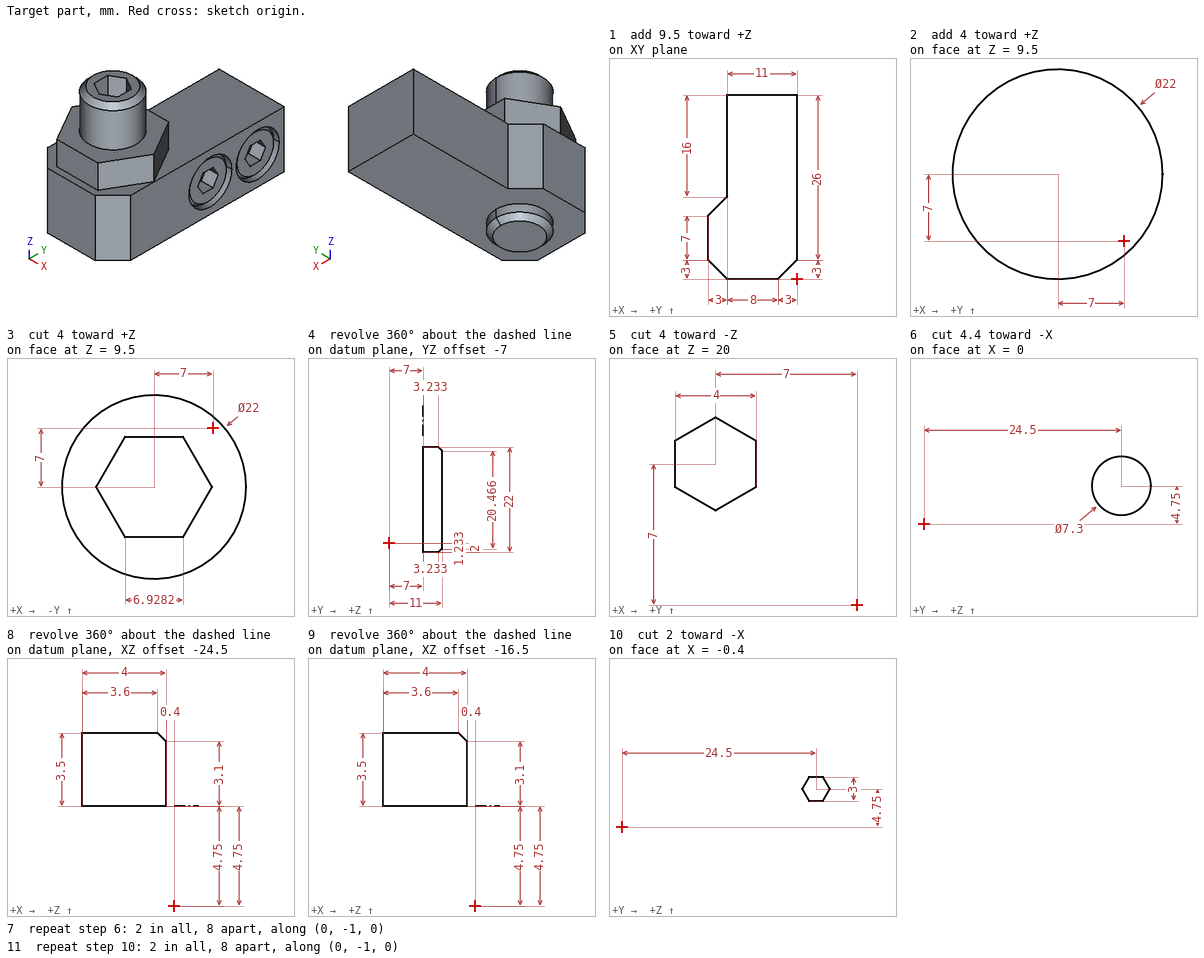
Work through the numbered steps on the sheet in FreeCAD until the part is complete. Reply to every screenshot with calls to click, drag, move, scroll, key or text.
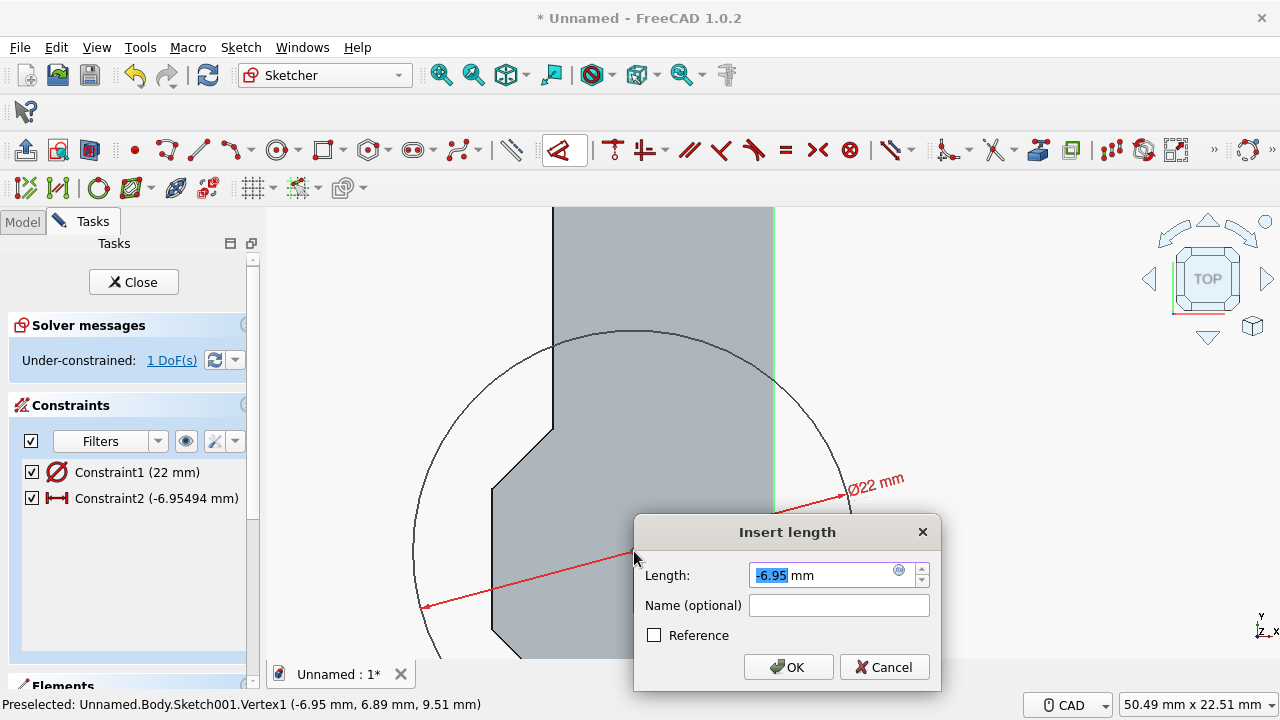
text(-7)
key(Return)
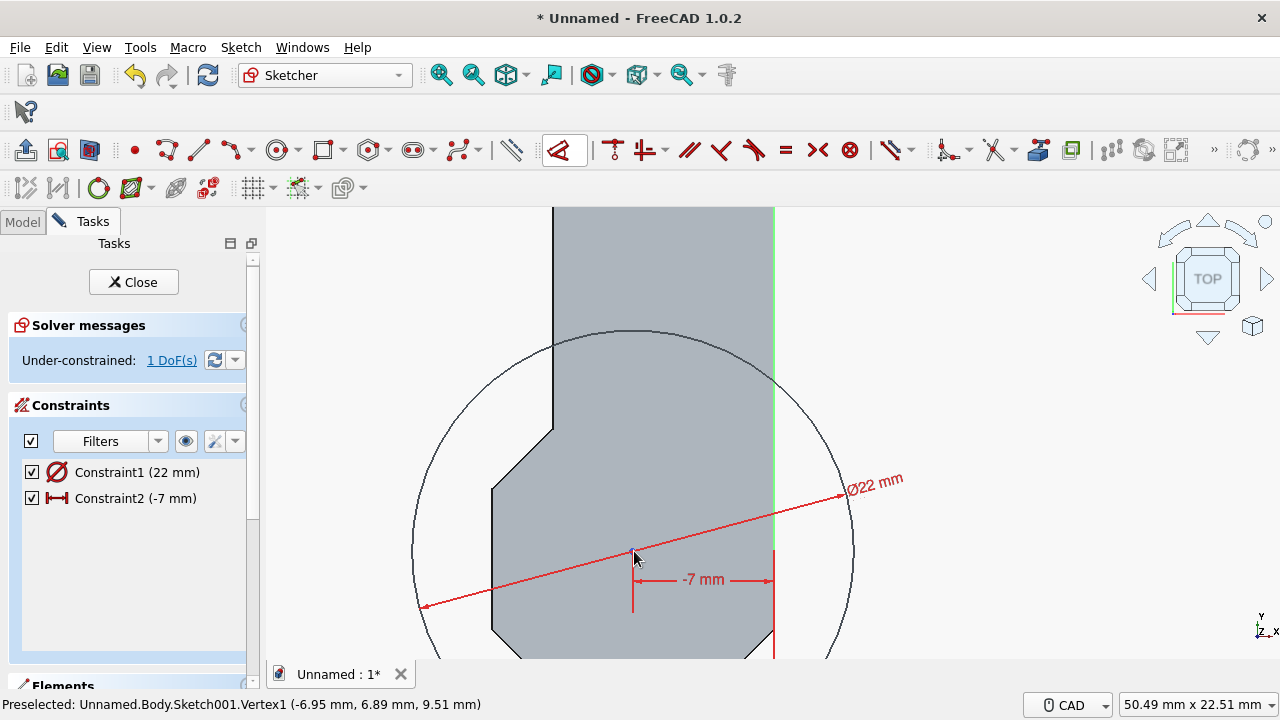
click(633, 551)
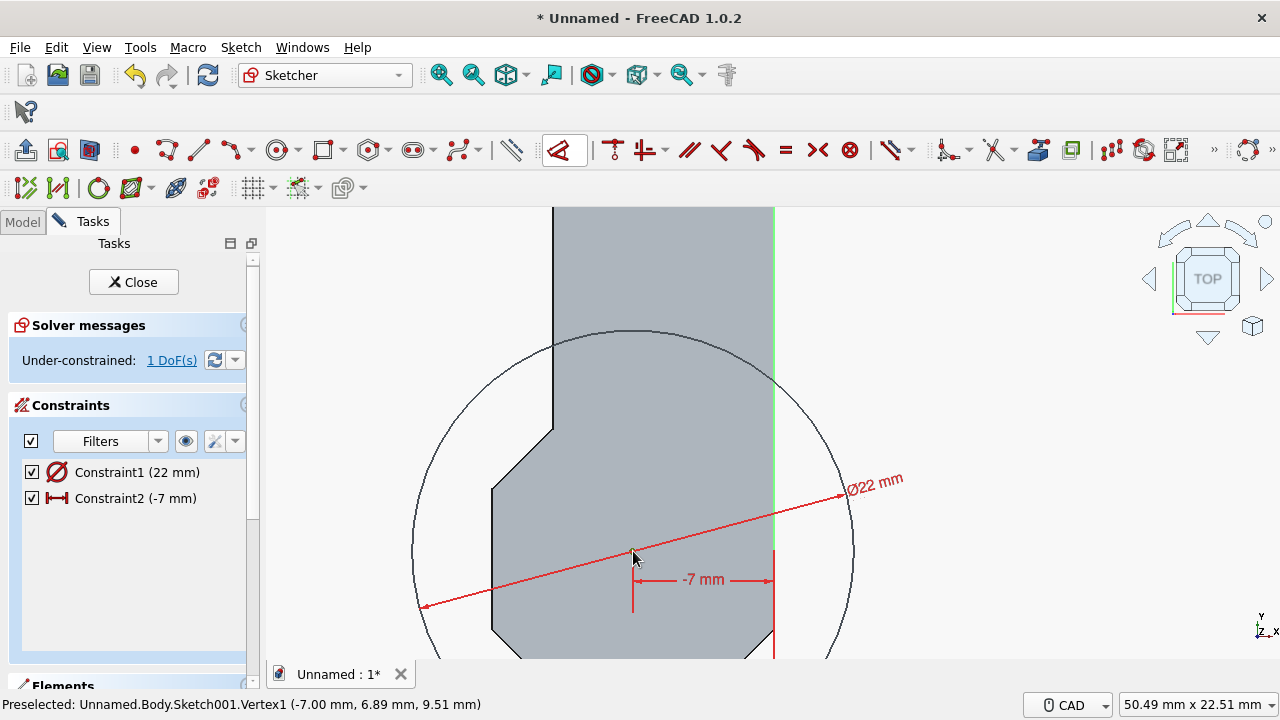
key(i)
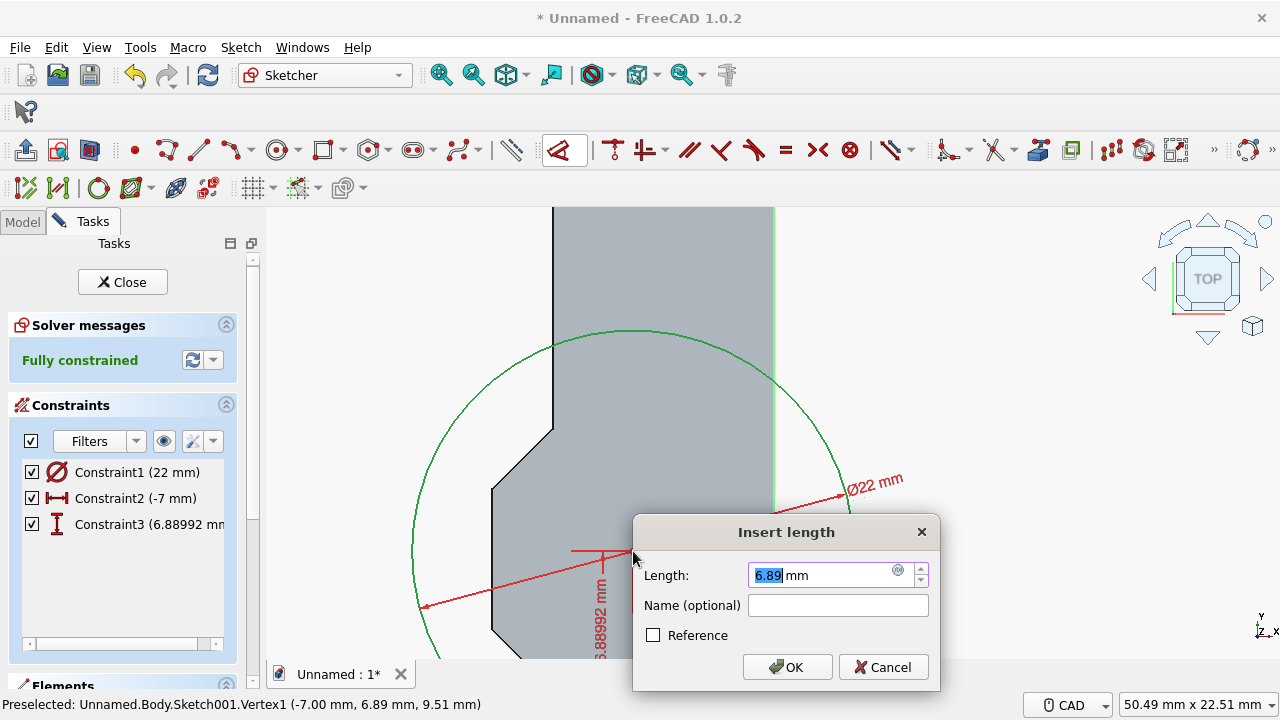
text(7)
key(Return)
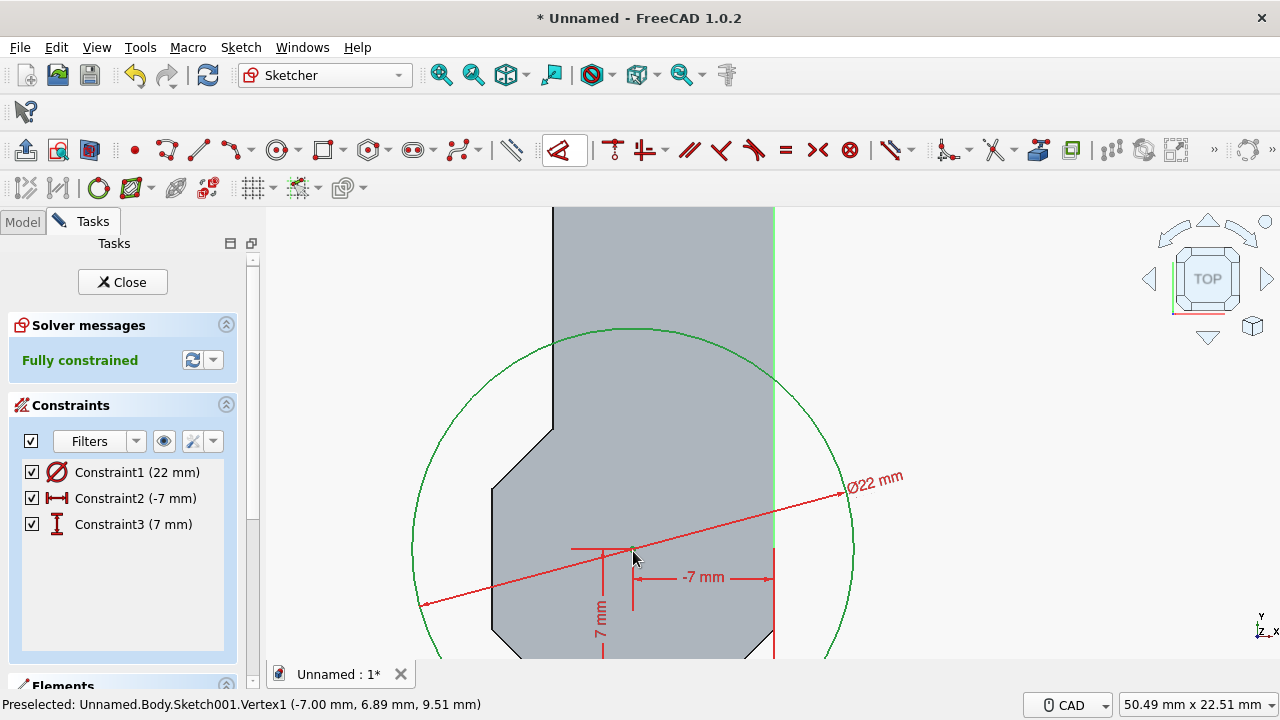
click(123, 282)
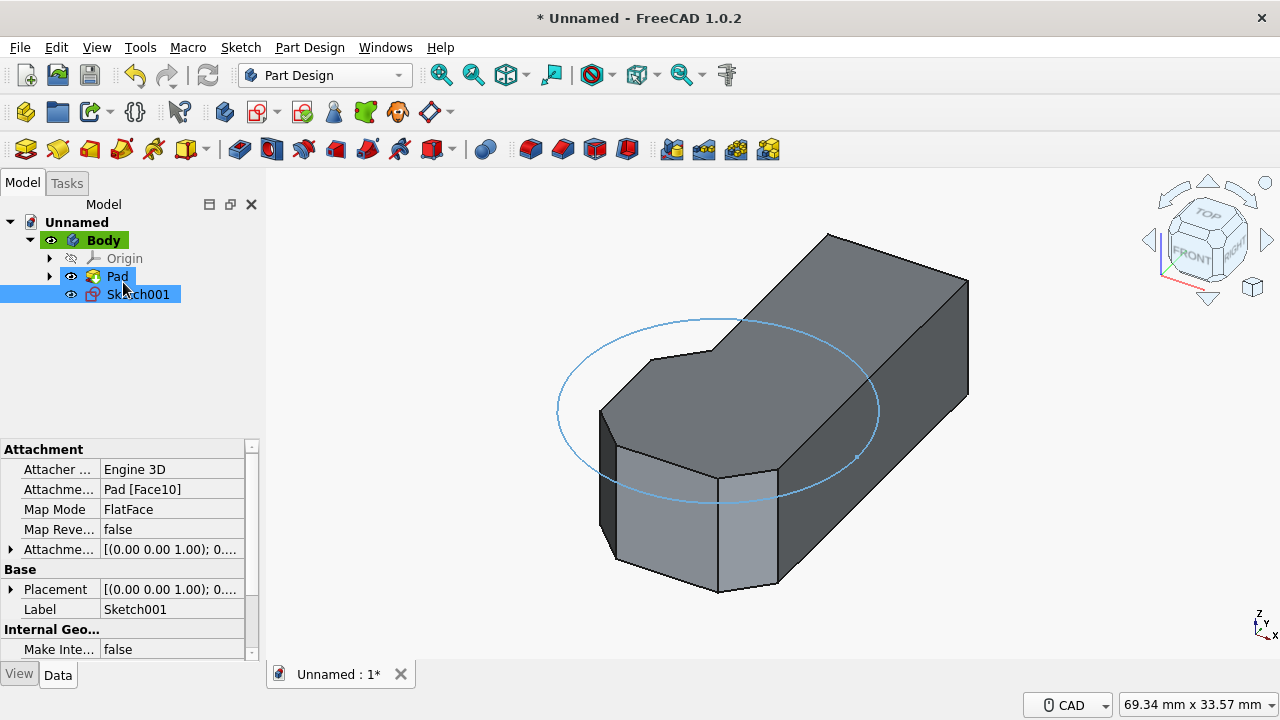
click(26, 150)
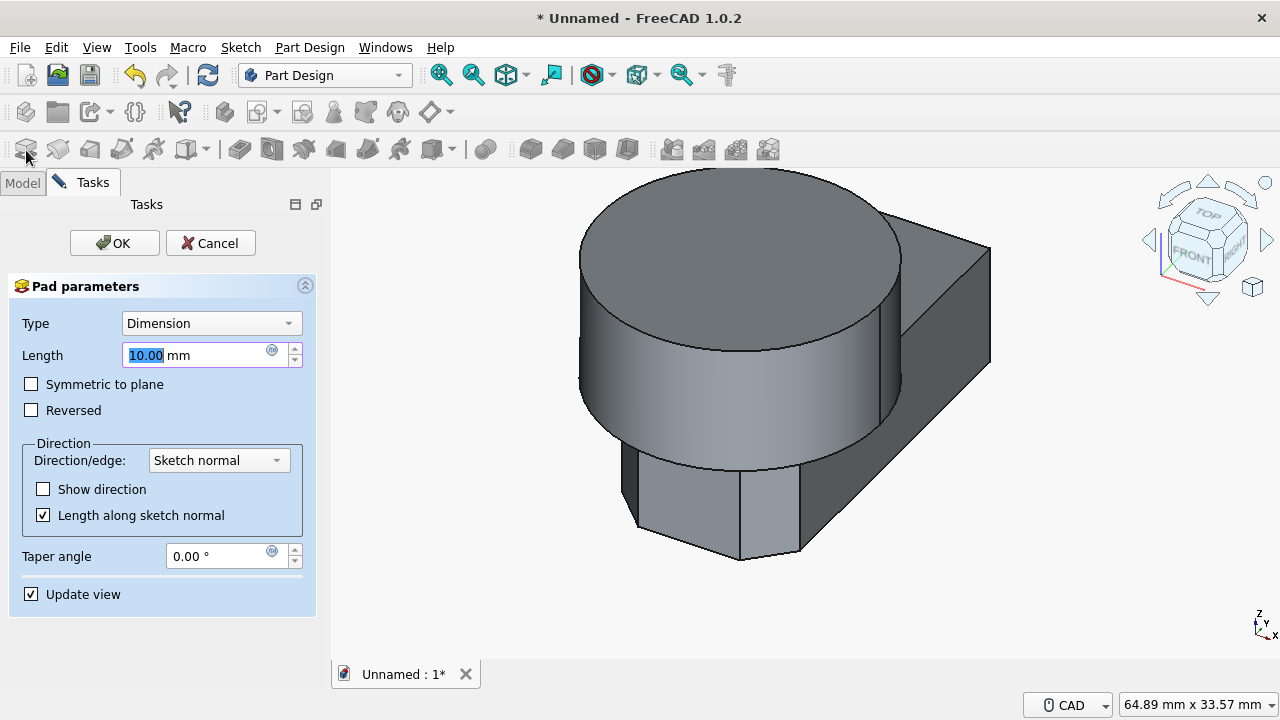
text(4)
key(Tab)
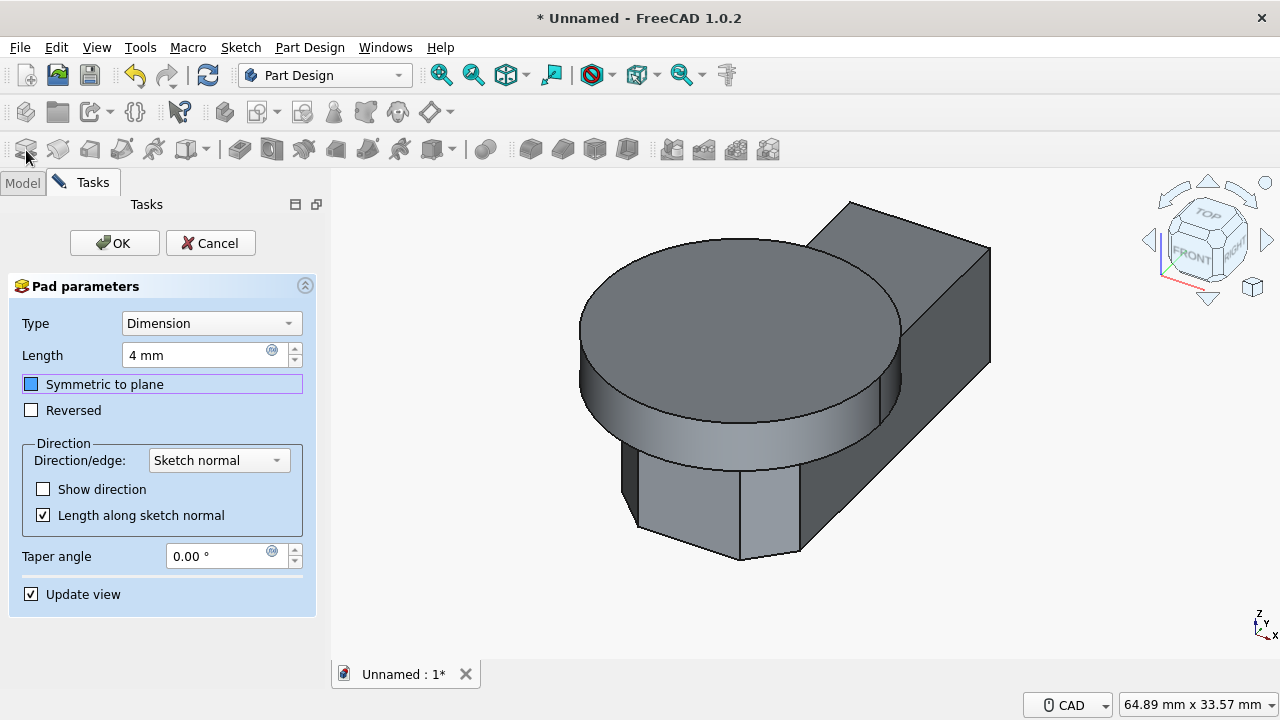
click(115, 243)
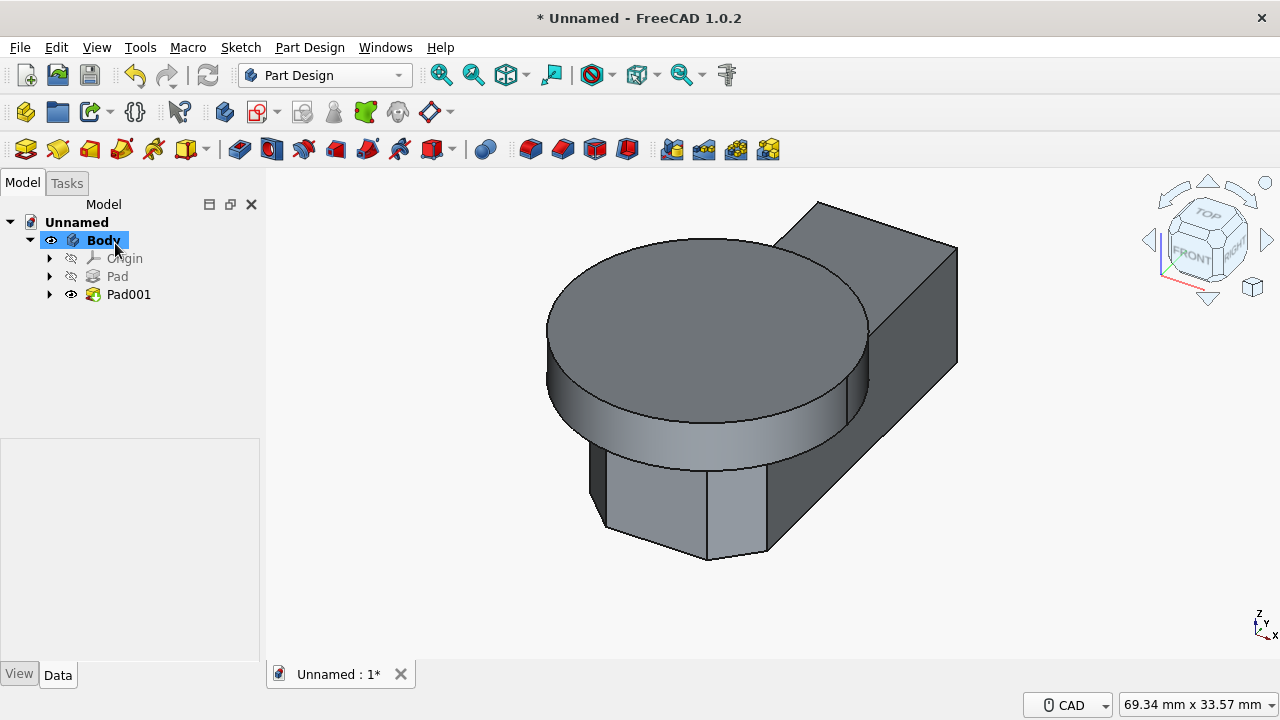
click(442, 76)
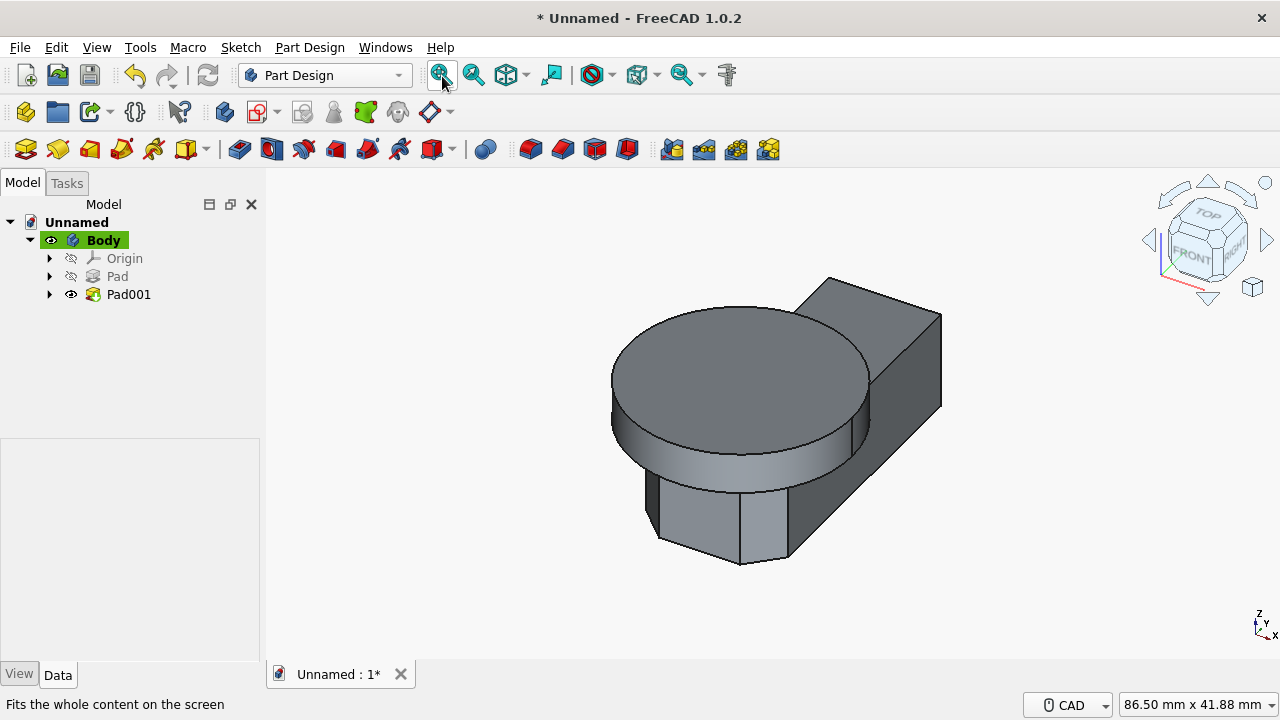
key(5)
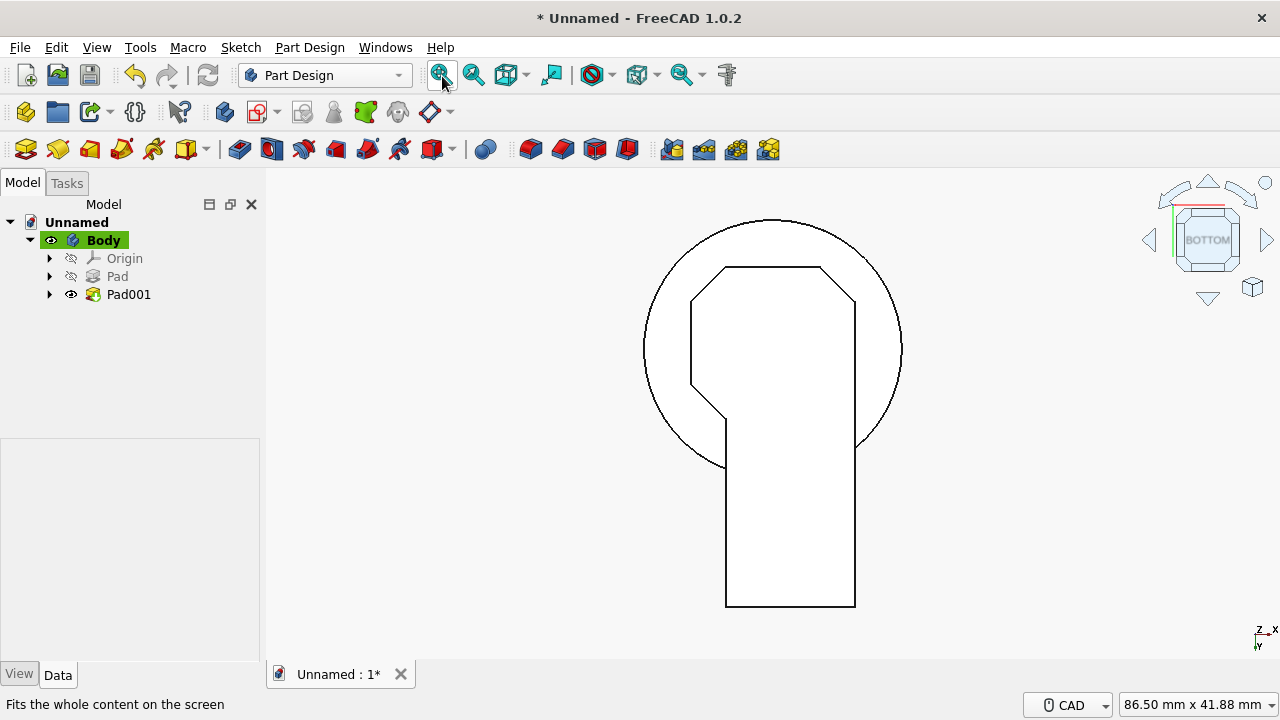
click(883, 344)